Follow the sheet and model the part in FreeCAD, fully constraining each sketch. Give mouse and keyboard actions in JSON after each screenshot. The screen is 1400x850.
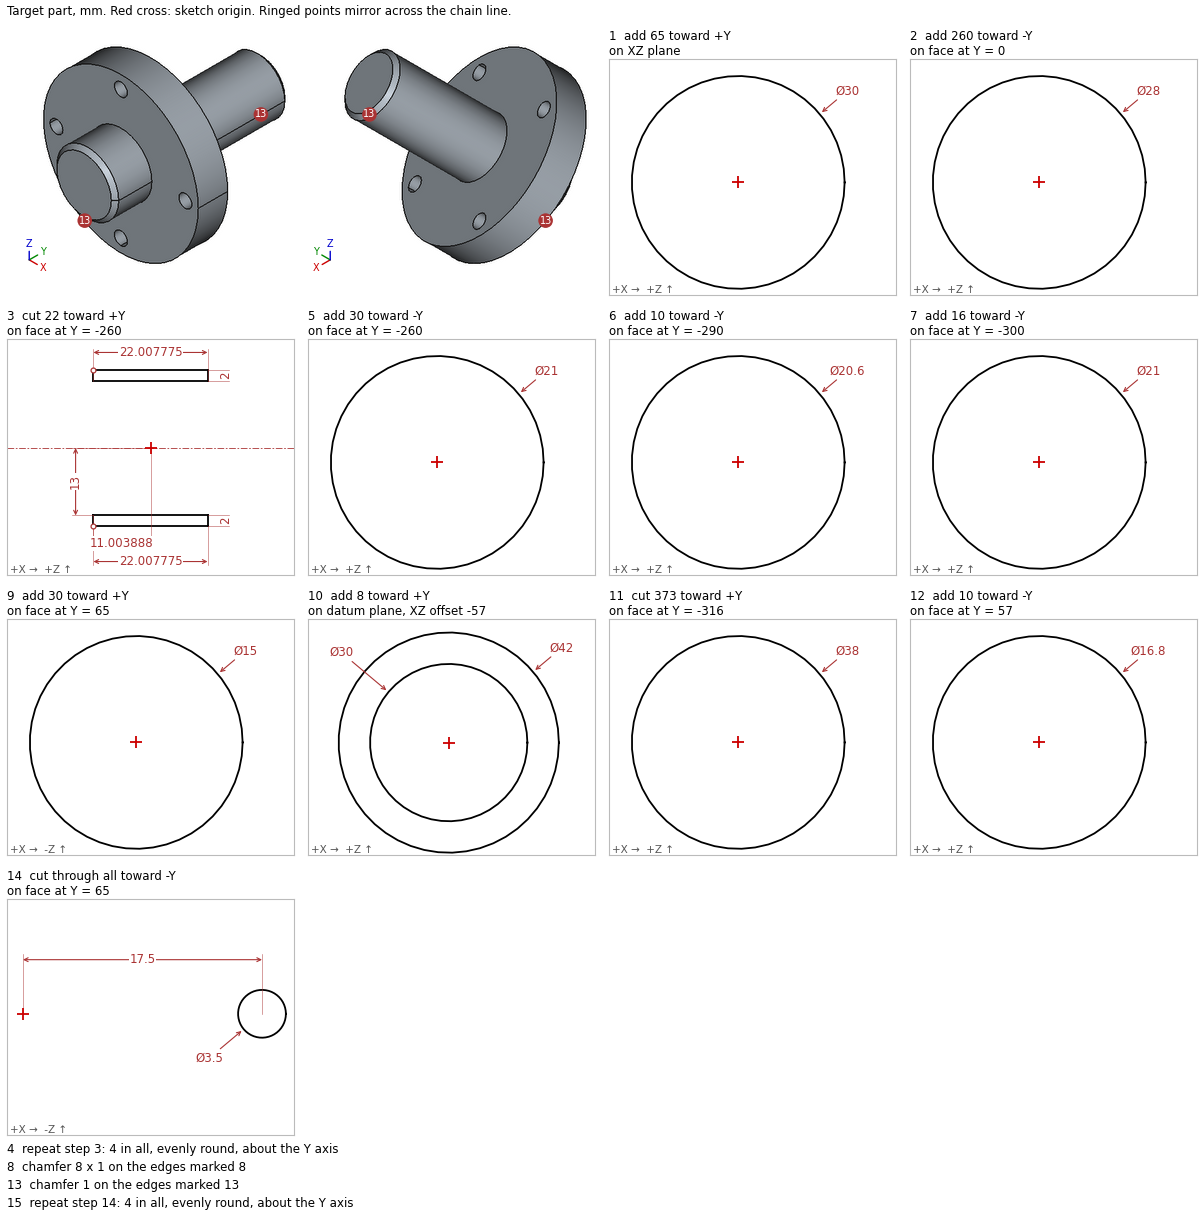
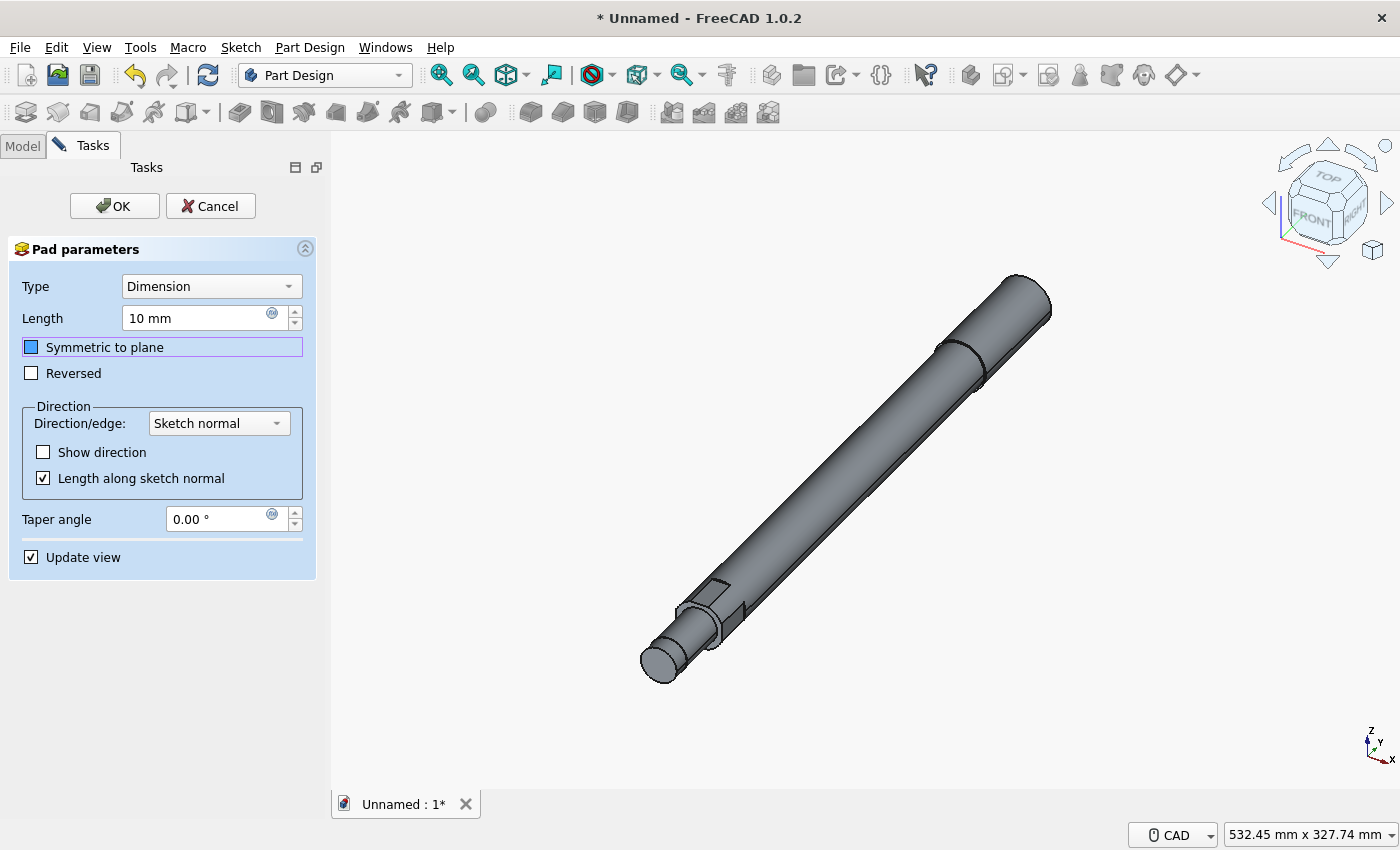
{"action": "left_click", "coordinate": [115, 206]}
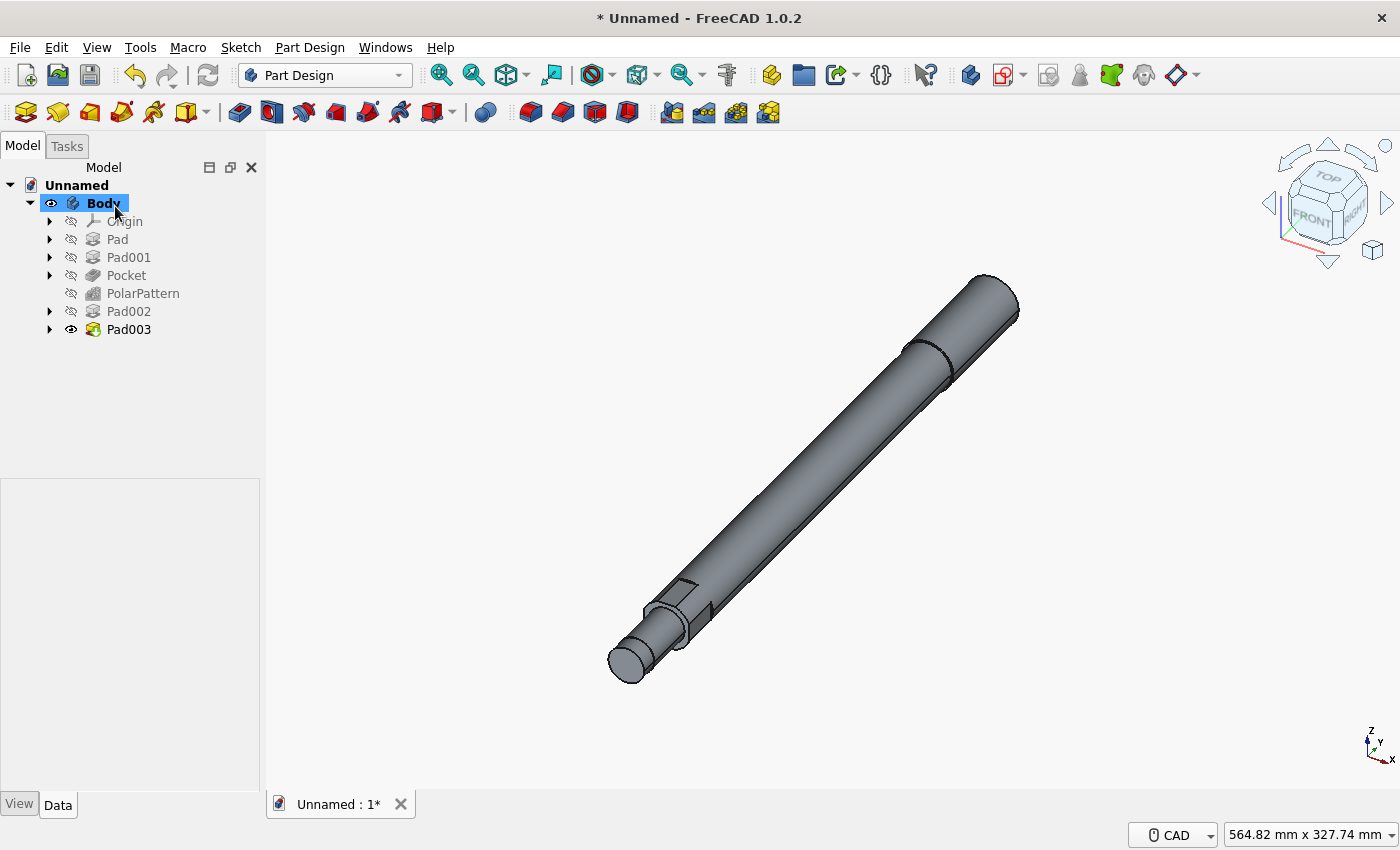
{"action": "left_click", "coordinate": [626, 664]}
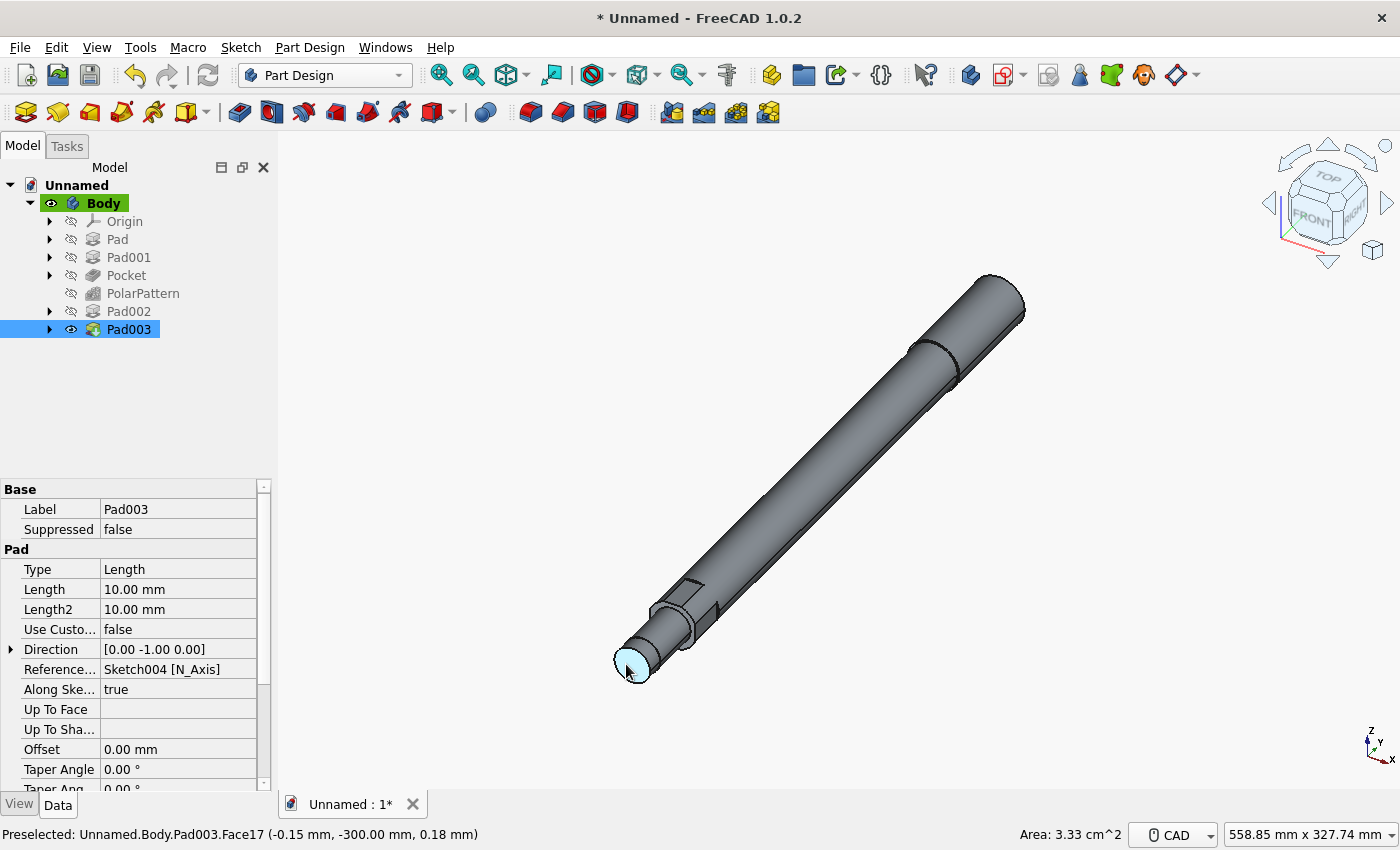
{"action": "left_click", "coordinate": [1004, 76]}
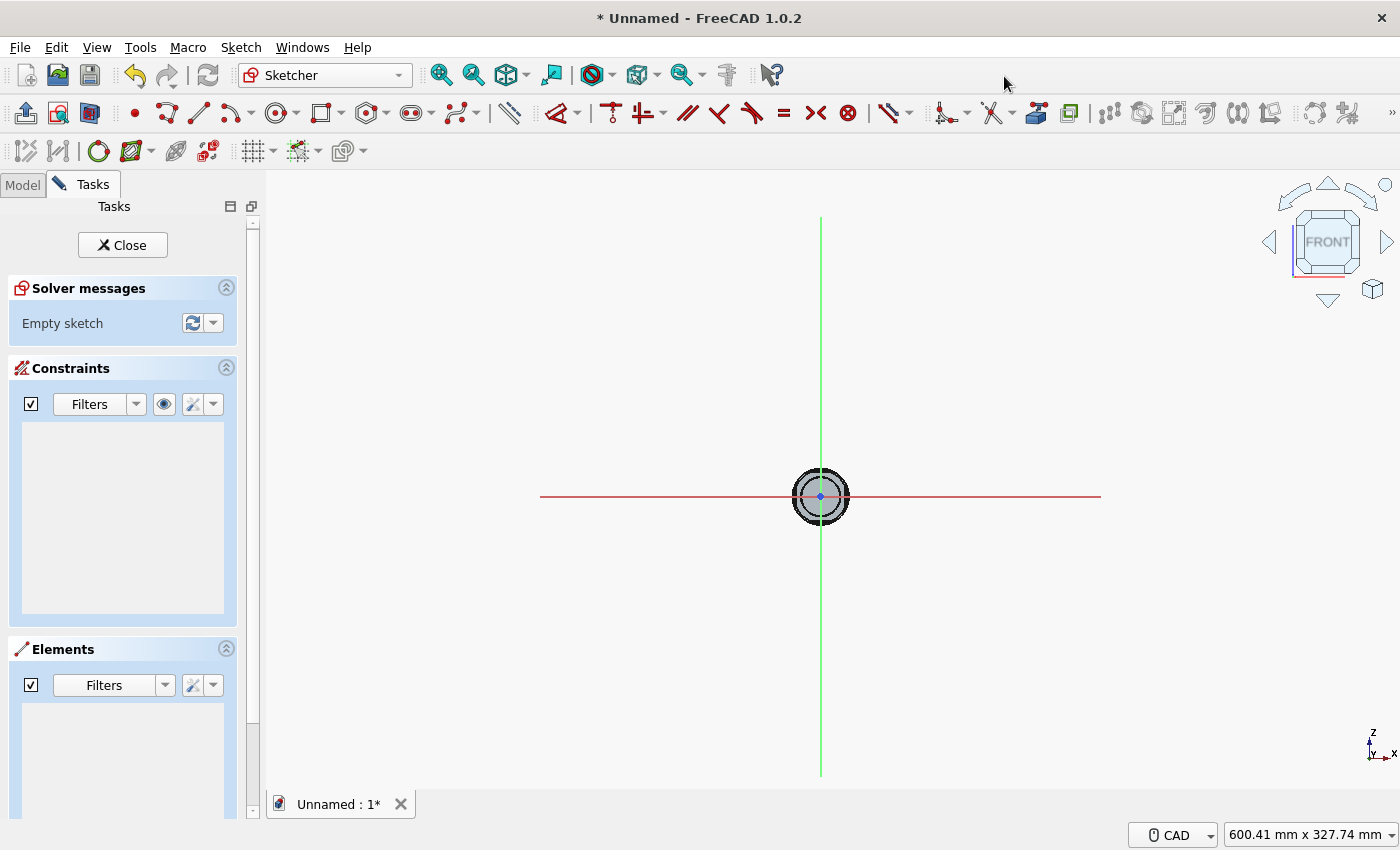
{"action": "scroll", "coordinate": [826, 498], "scroll_direction": "up", "scroll_amount": 12}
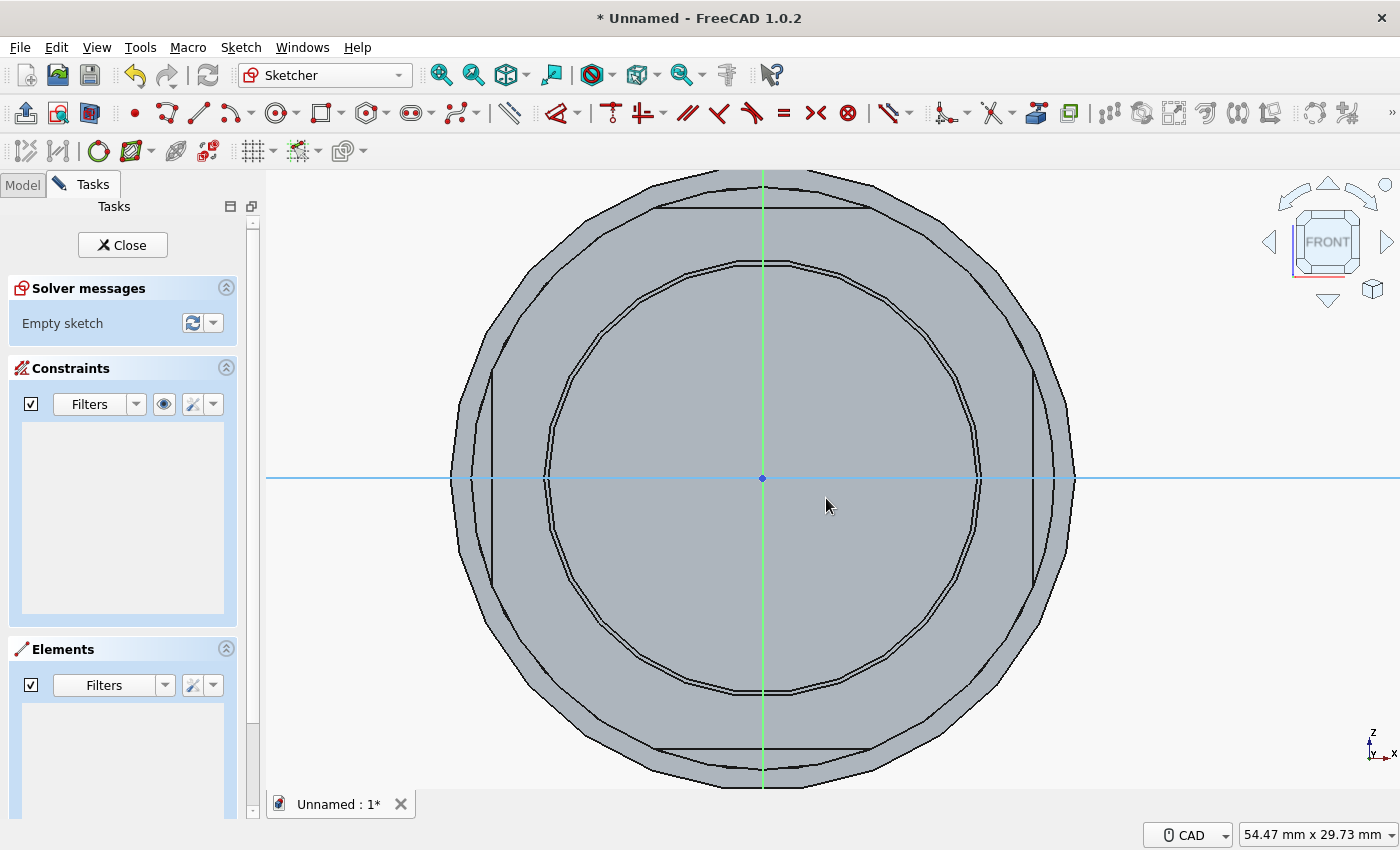
{"action": "left_click", "coordinate": [276, 114]}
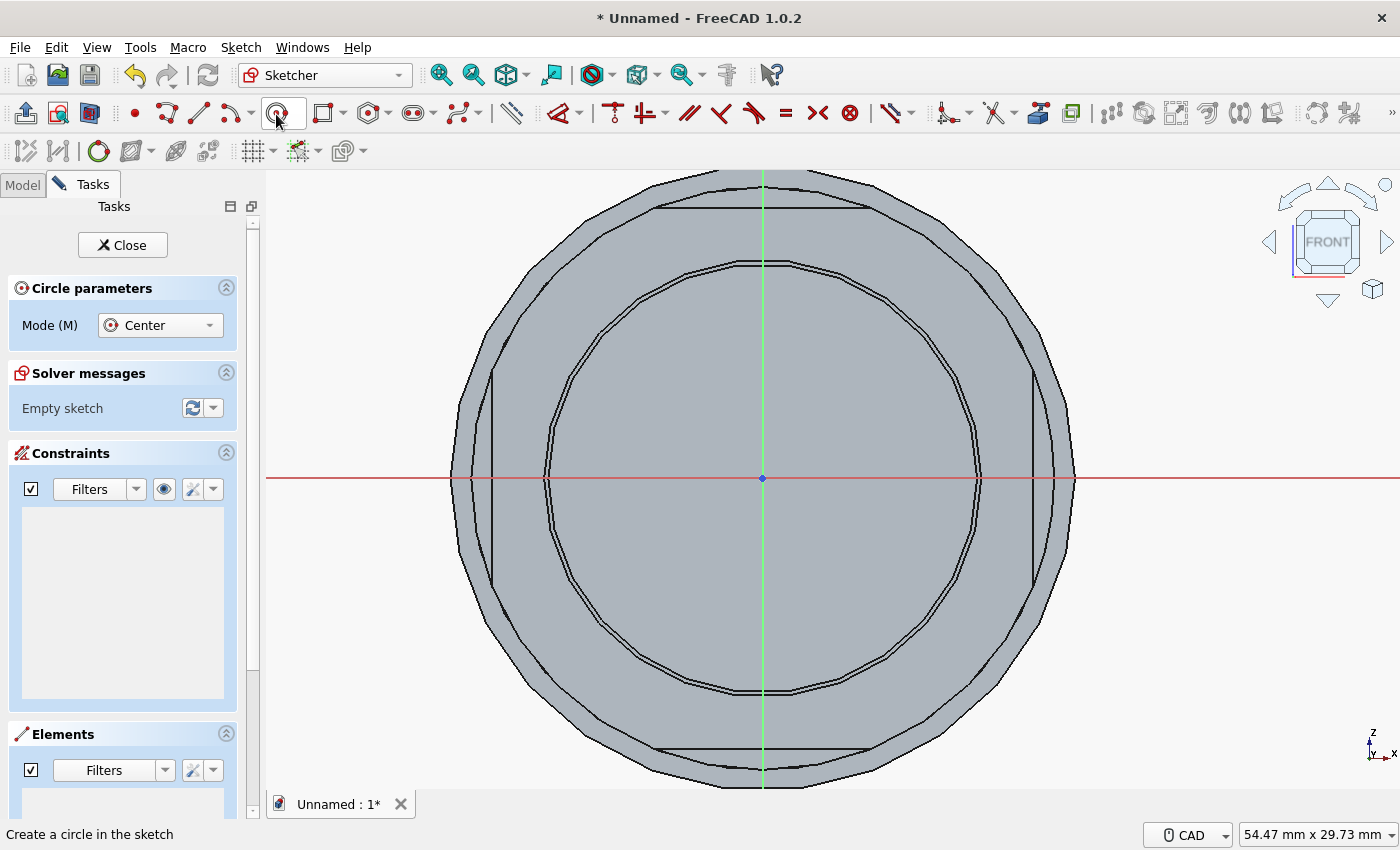
{"action": "left_click", "coordinate": [763, 478]}
{"action": "mouse_move", "coordinate": [917, 324]}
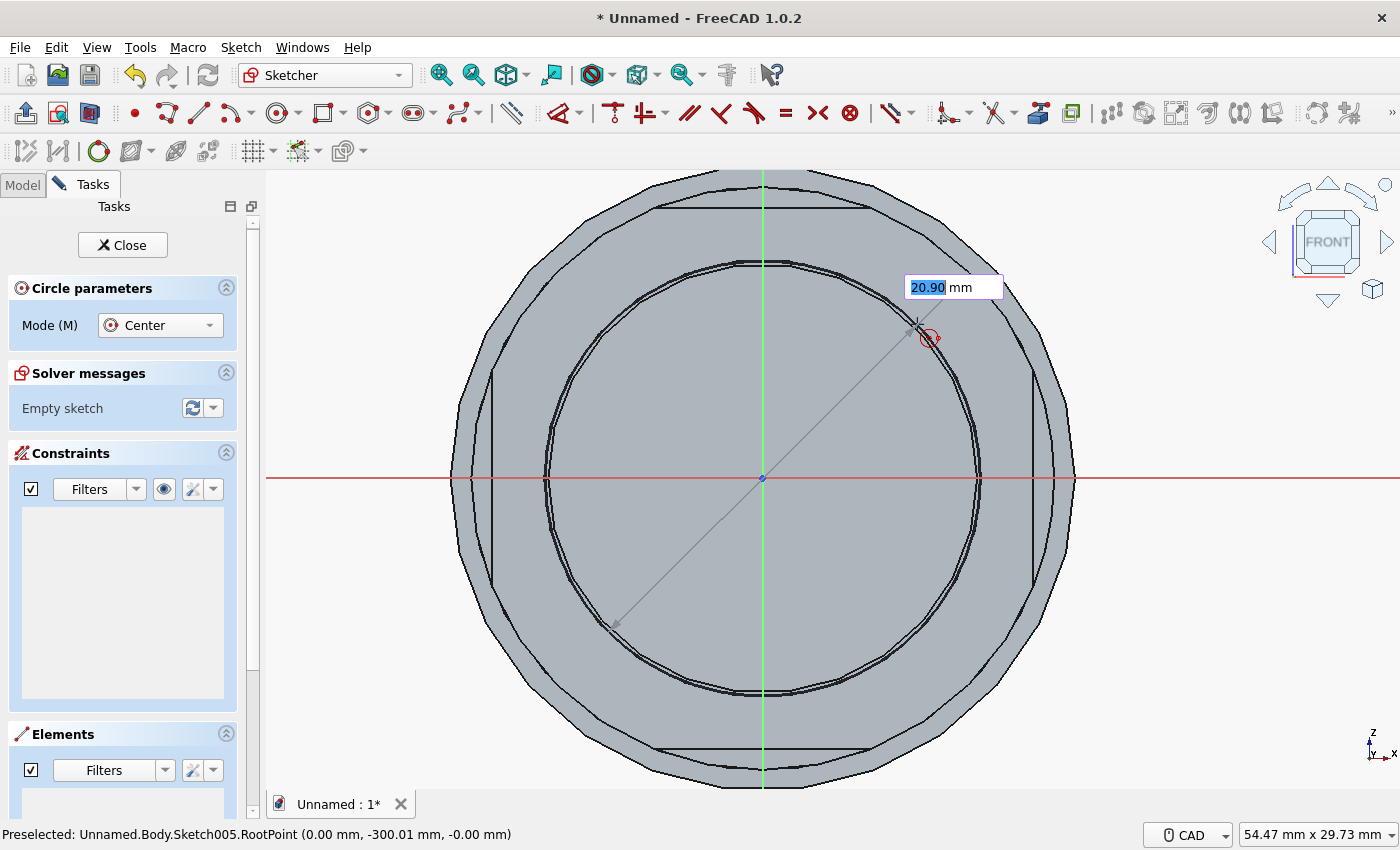
{"action": "type", "text": "21"}
{"action": "key", "text": "Return"}
{"action": "key", "text": "Escape"}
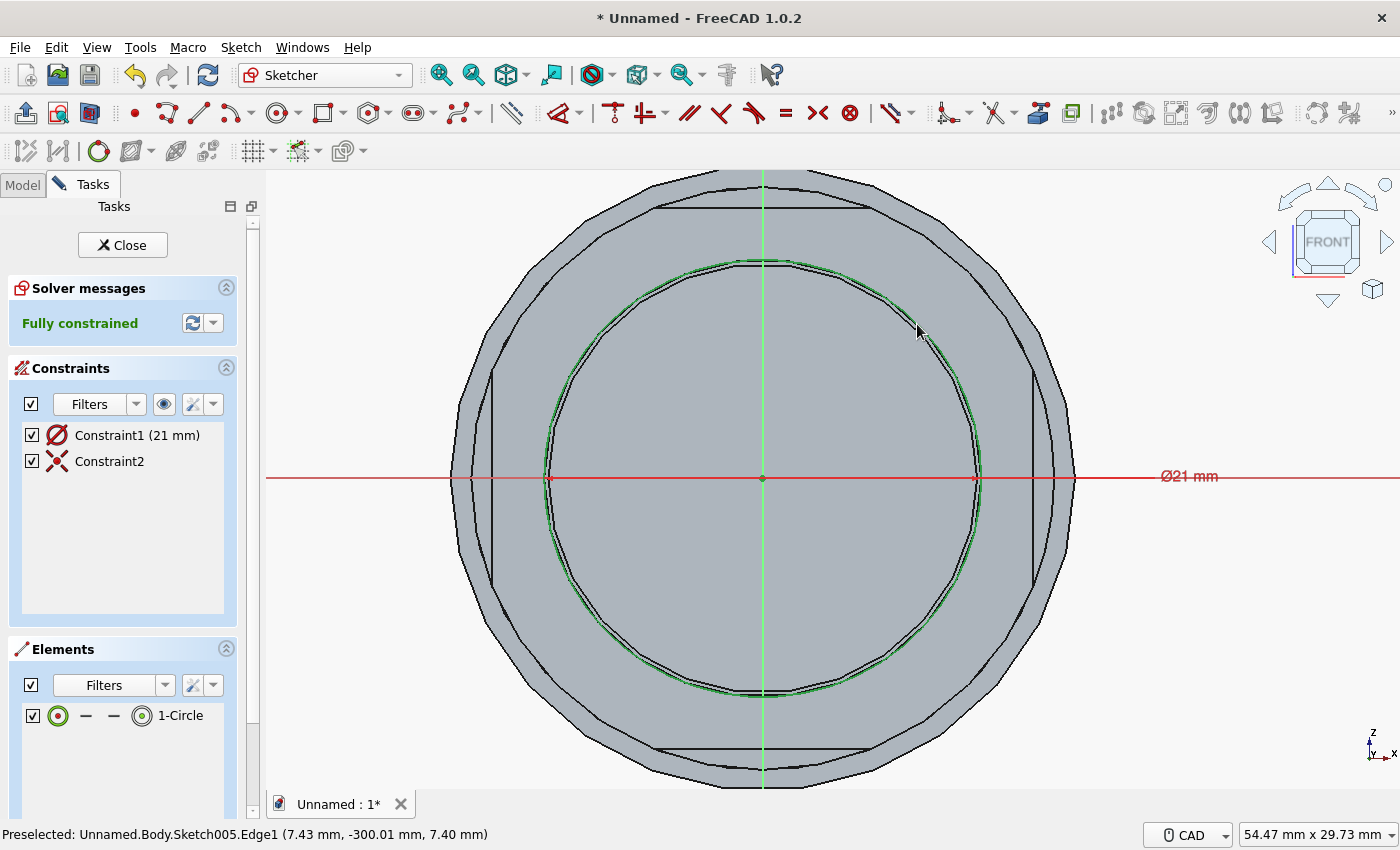
{"action": "left_click", "coordinate": [123, 245]}